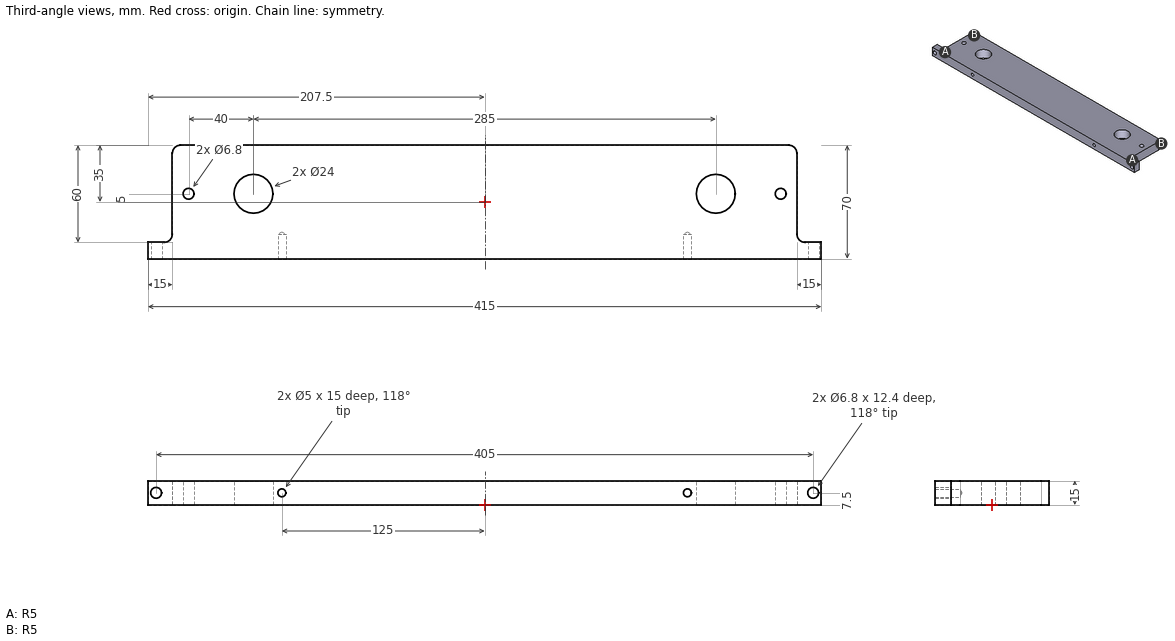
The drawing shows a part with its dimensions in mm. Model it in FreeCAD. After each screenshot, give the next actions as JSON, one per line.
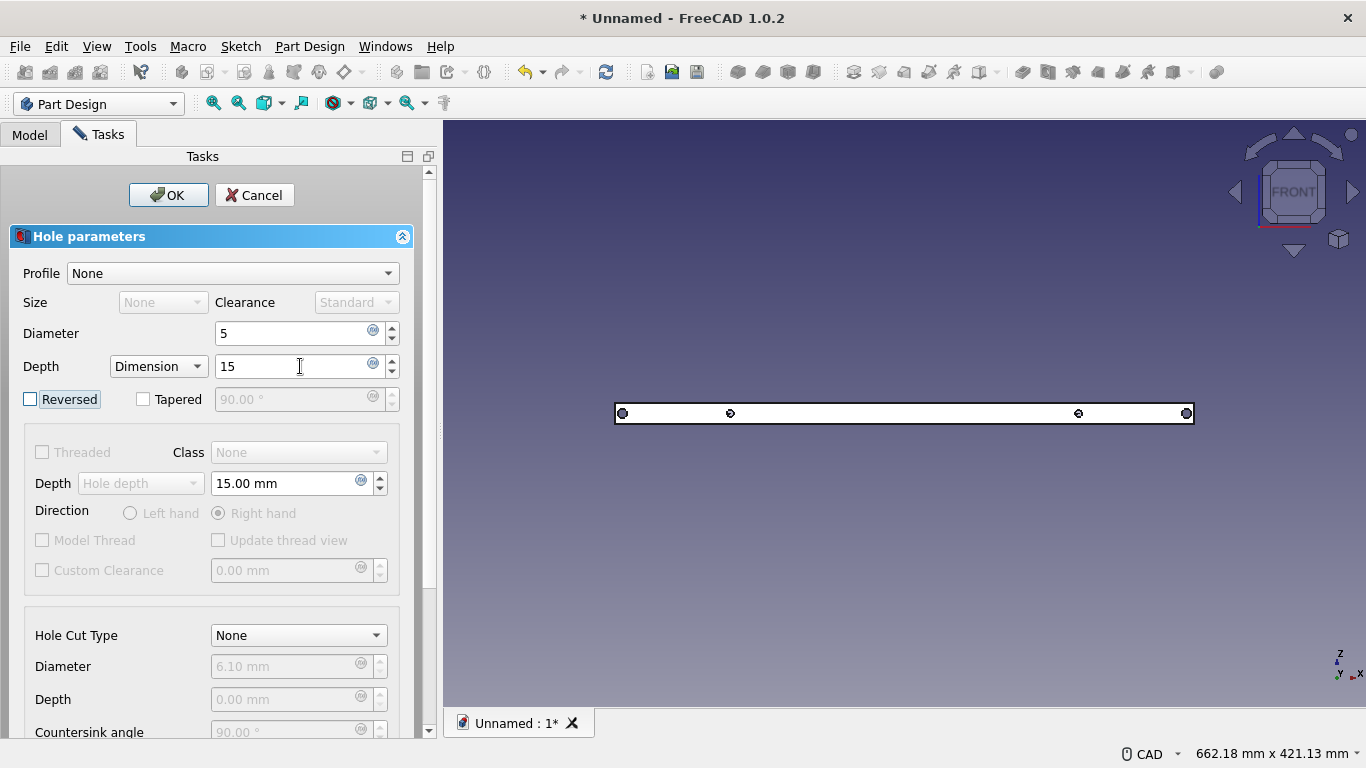
{"action": "left_click", "coordinate": [169, 195]}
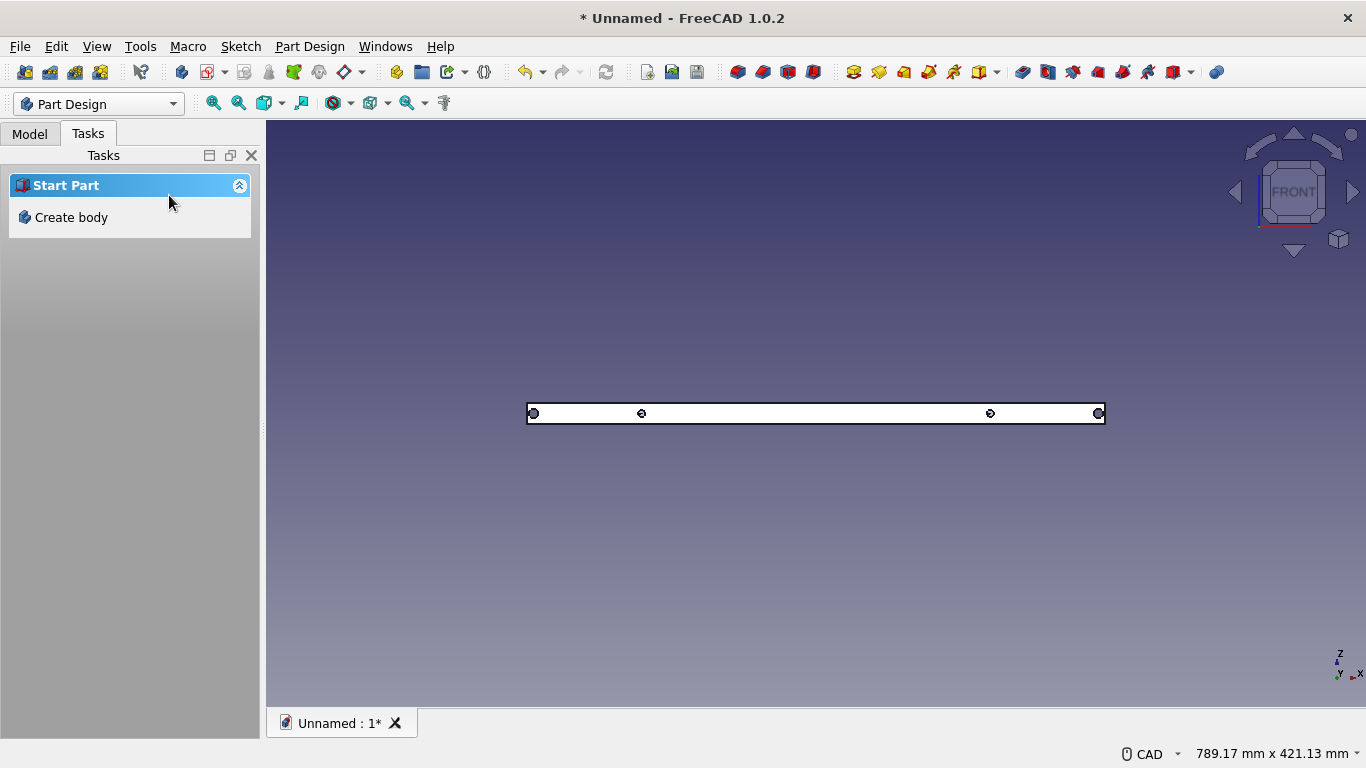
{"action": "key", "text": "0"}